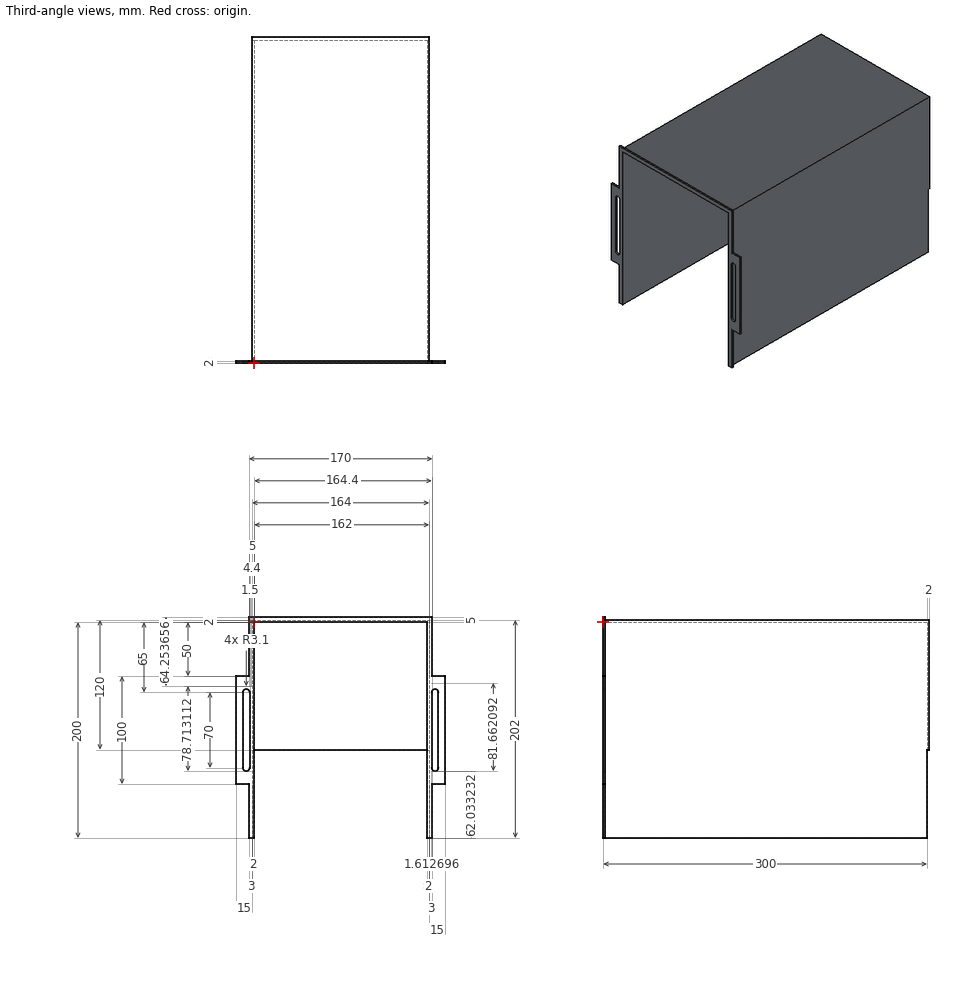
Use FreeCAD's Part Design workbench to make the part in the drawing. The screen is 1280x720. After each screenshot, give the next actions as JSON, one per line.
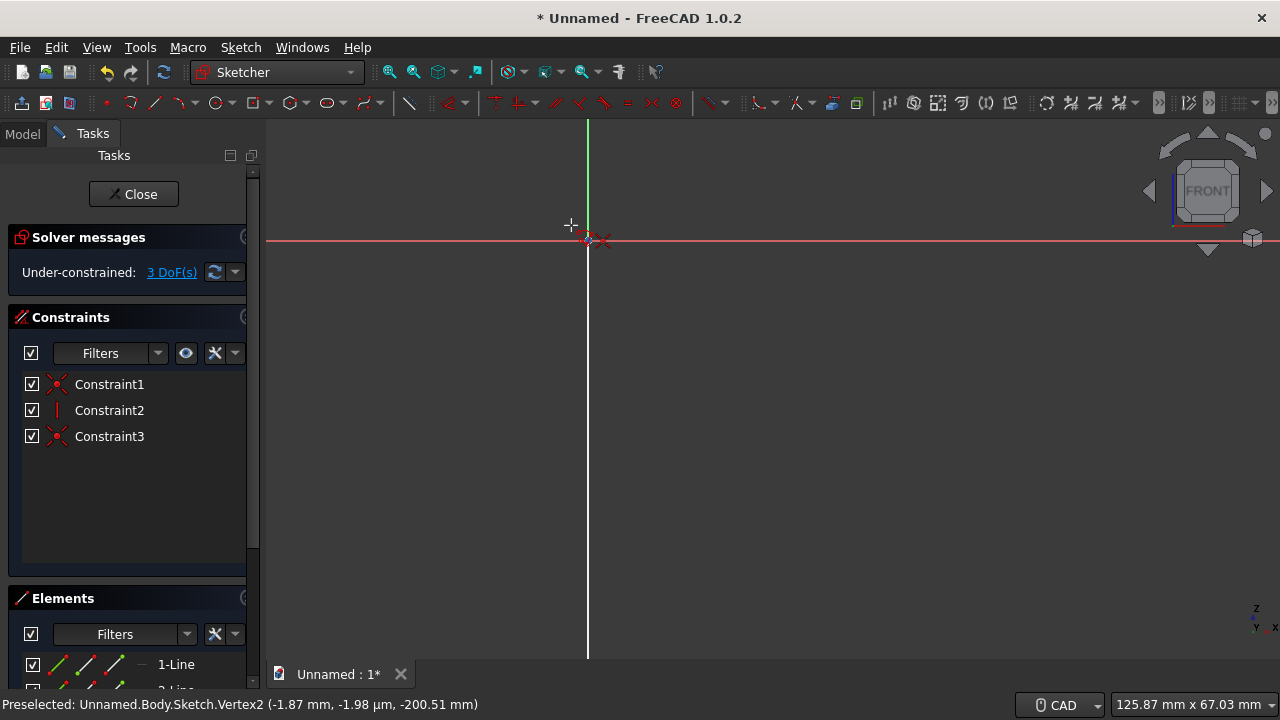
{"action": "left_click", "coordinate": [572, 225]}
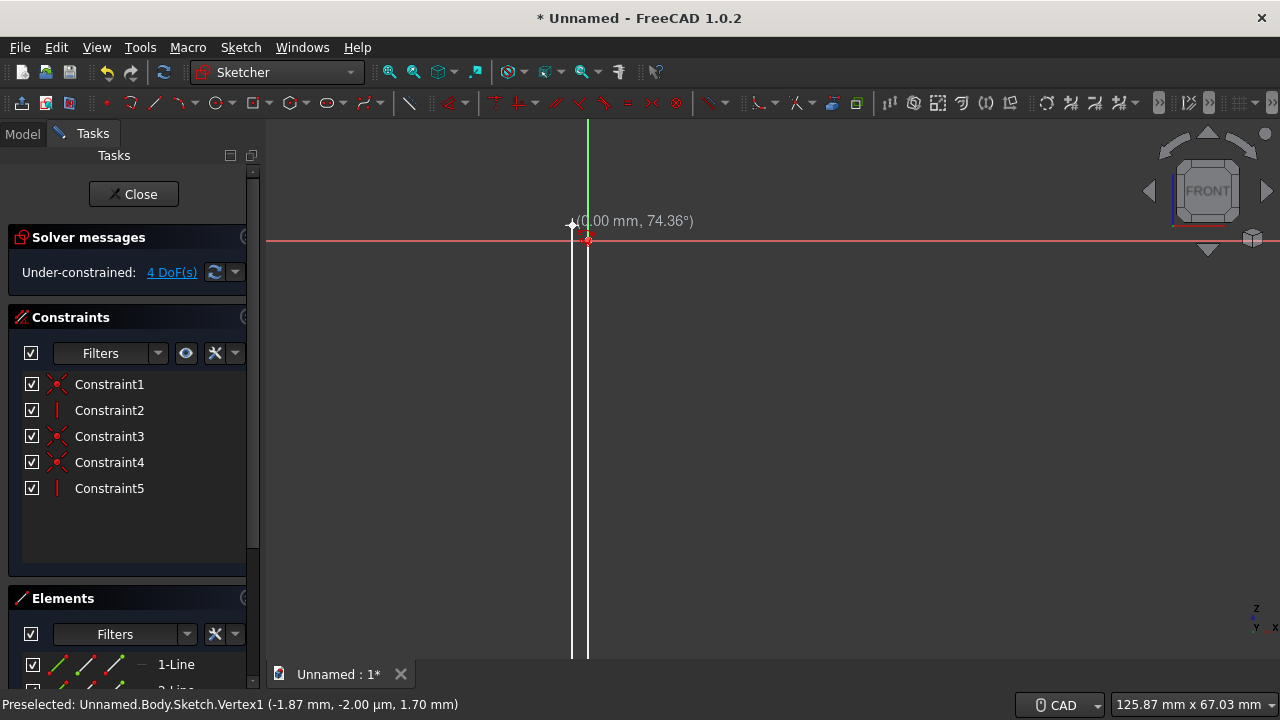
{"action": "scroll", "coordinate": [571, 225], "scroll_direction": "down", "scroll_amount": 8}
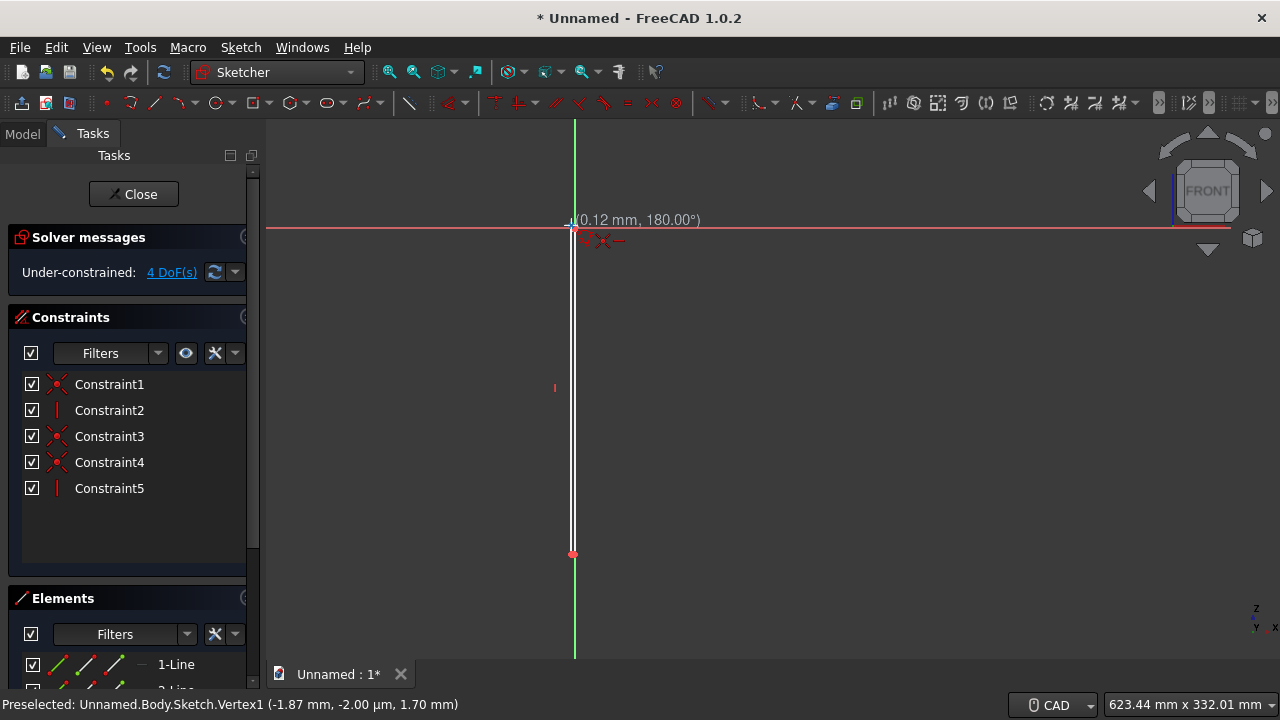
{"action": "scroll", "coordinate": [838, 225], "scroll_direction": "up", "scroll_amount": 8}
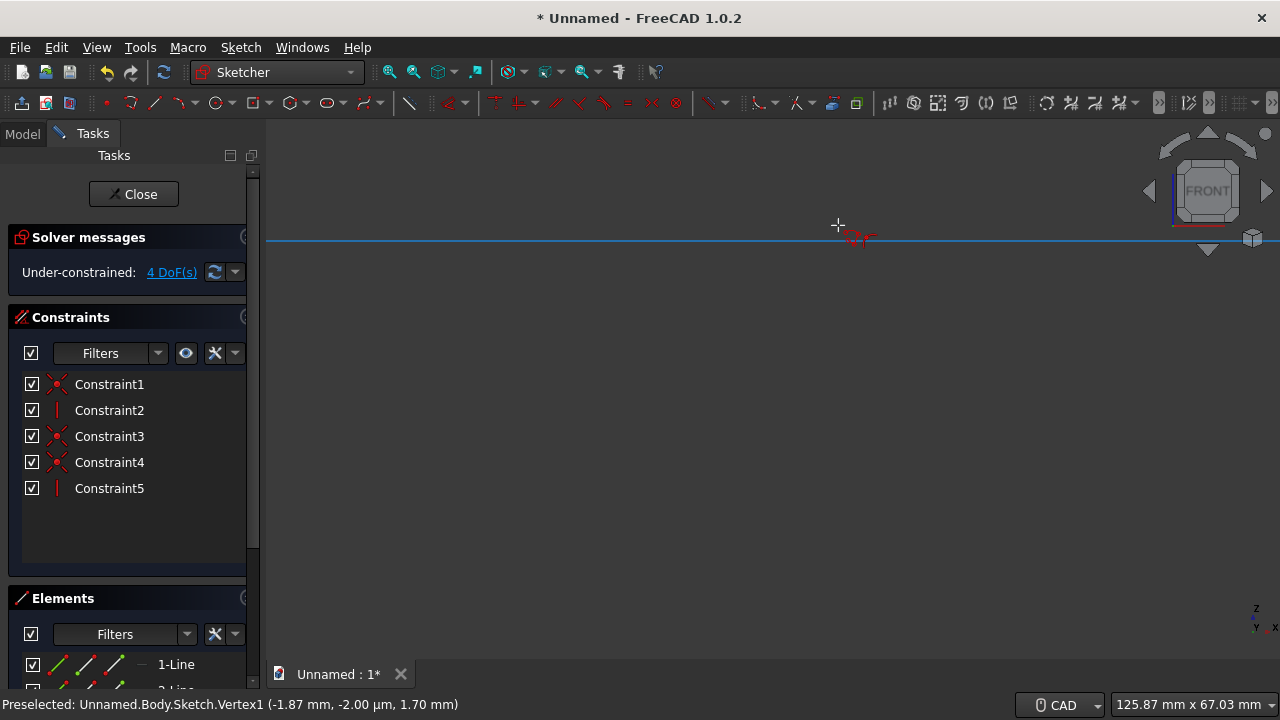
{"action": "left_click", "coordinate": [837, 225]}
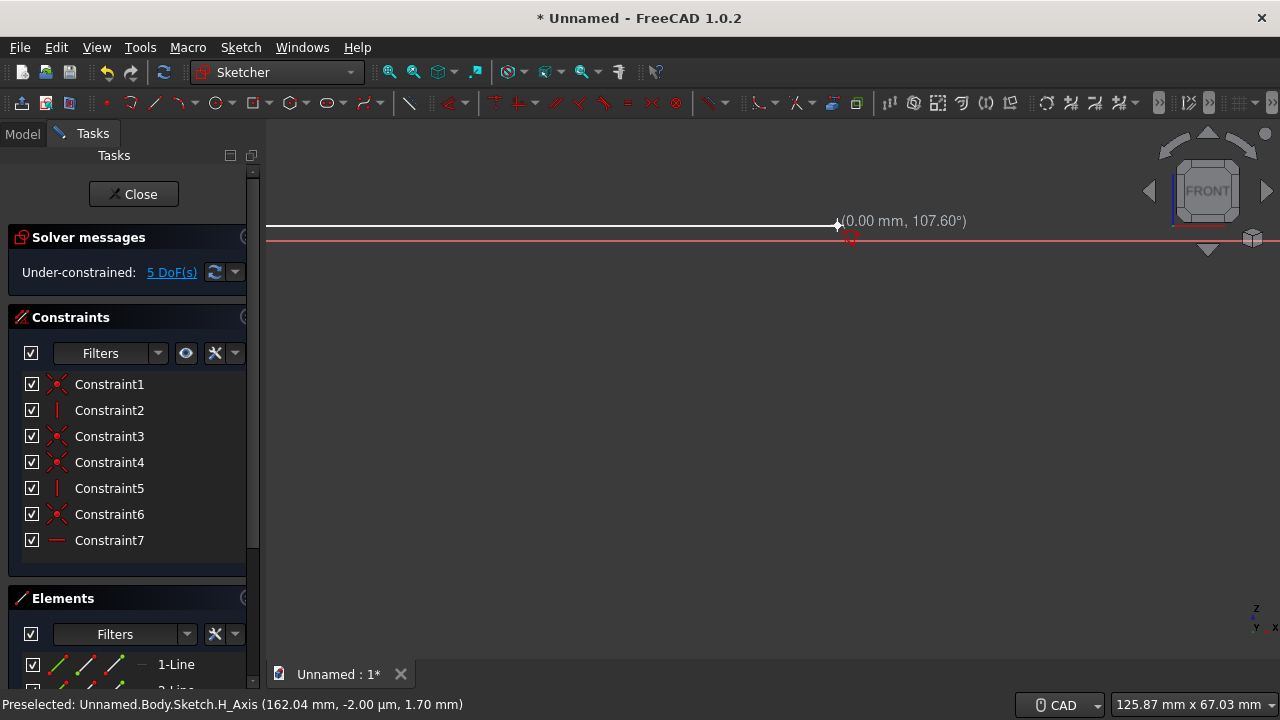
{"action": "scroll", "coordinate": [838, 225], "scroll_direction": "down", "scroll_amount": 8}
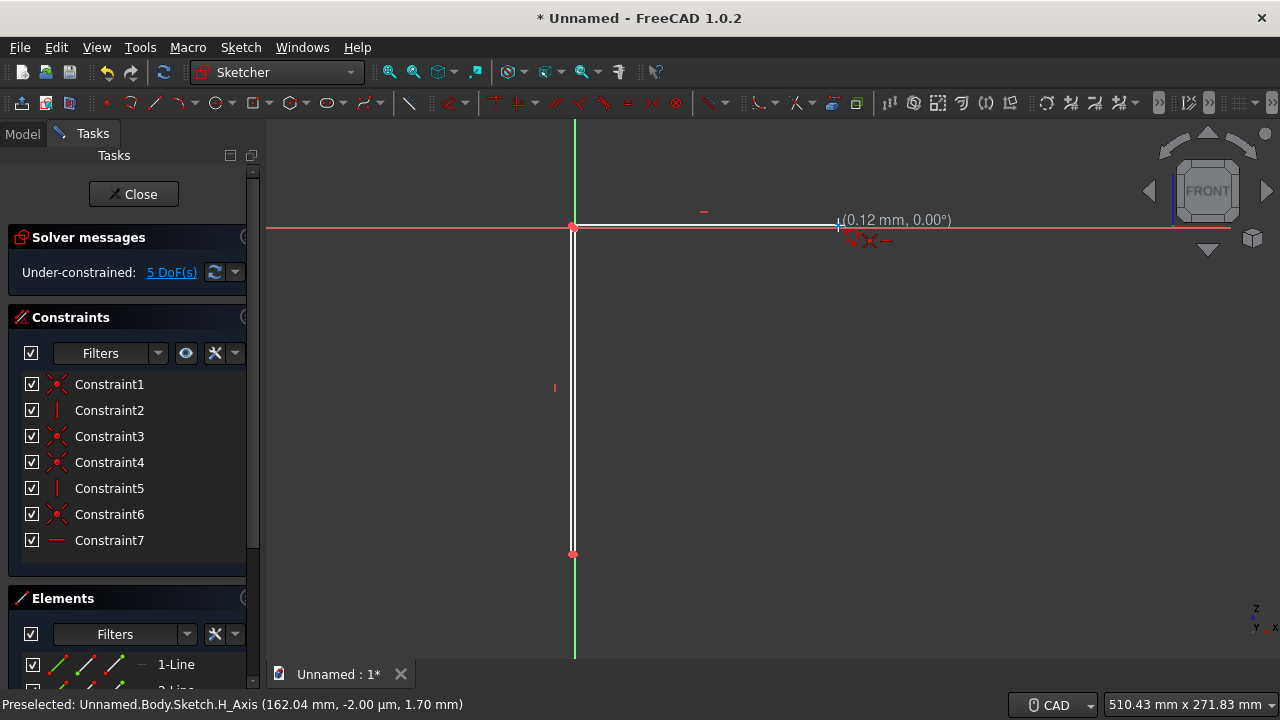
{"action": "left_click", "coordinate": [838, 554]}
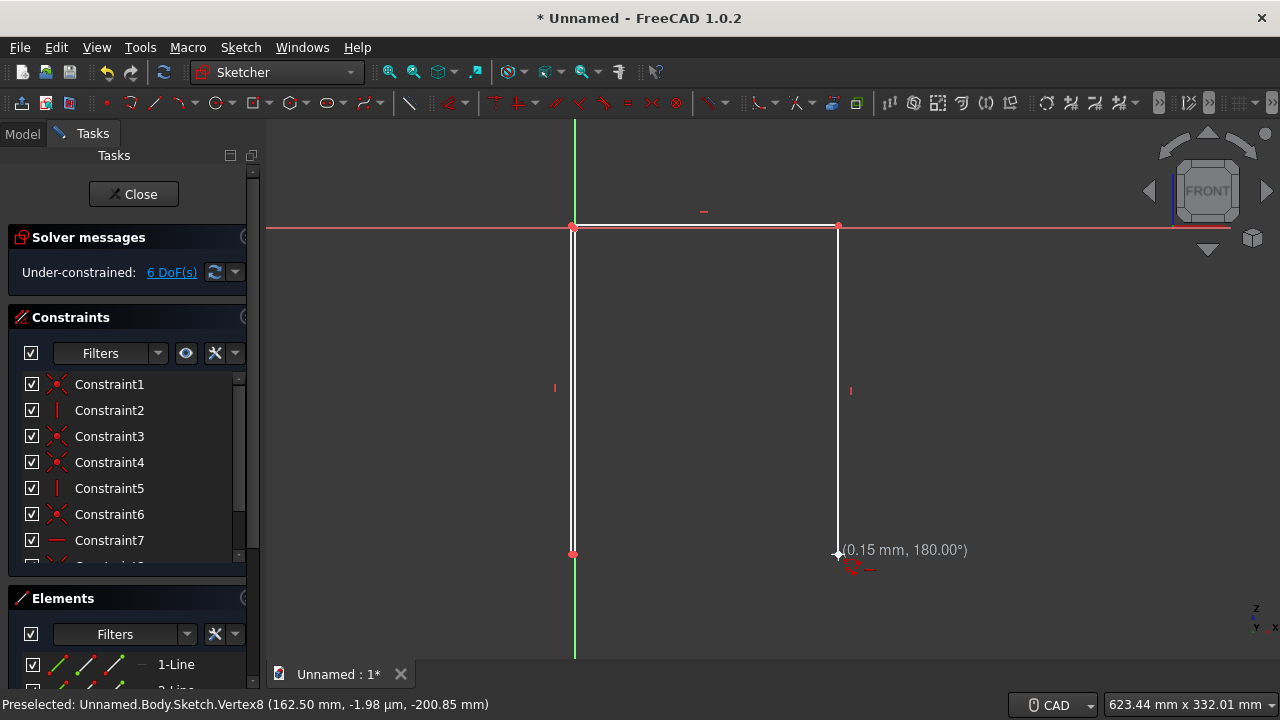
{"action": "scroll", "coordinate": [835, 554], "scroll_direction": "up", "scroll_amount": 8}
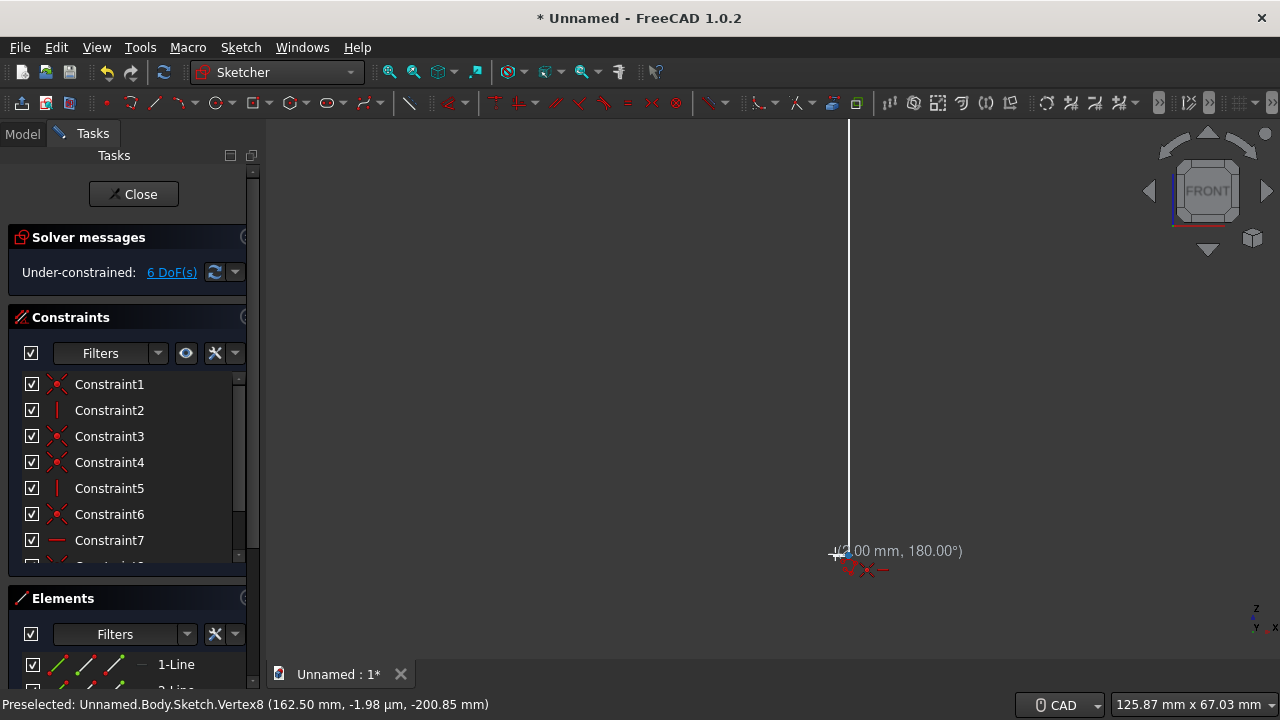
{"action": "left_click", "coordinate": [832, 551]}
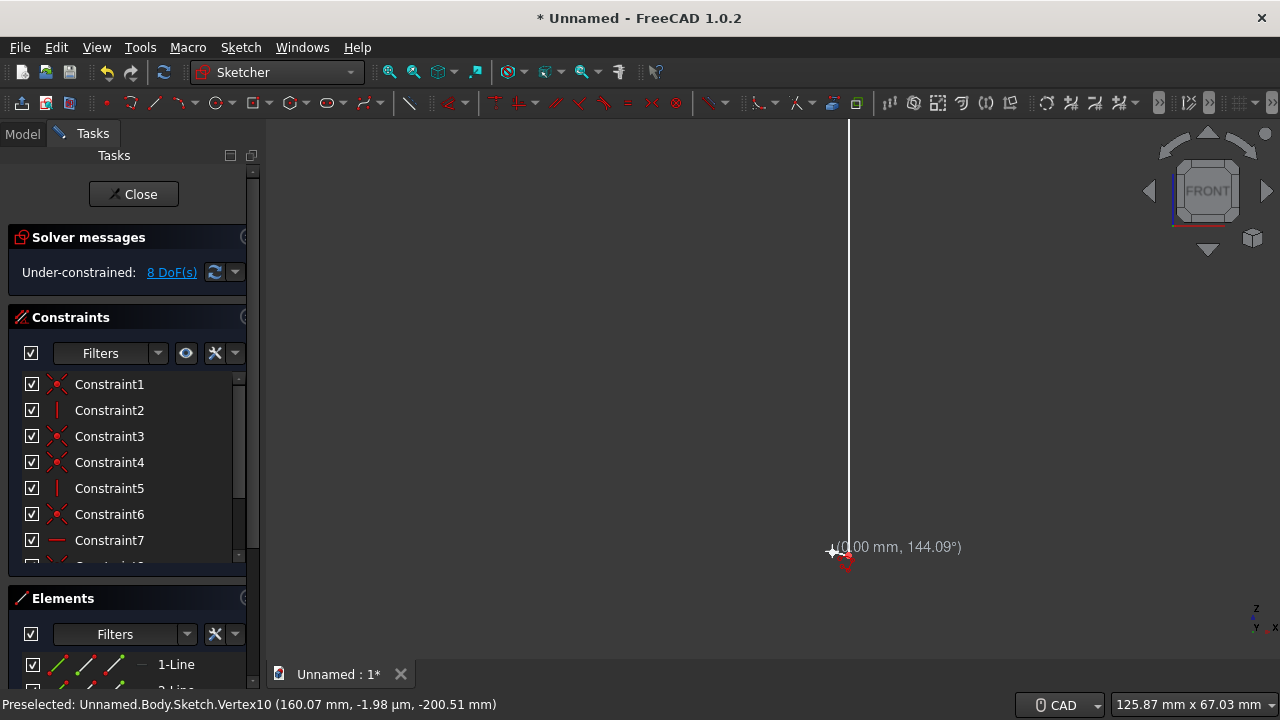
{"action": "scroll", "coordinate": [835, 554], "scroll_direction": "down", "scroll_amount": 8}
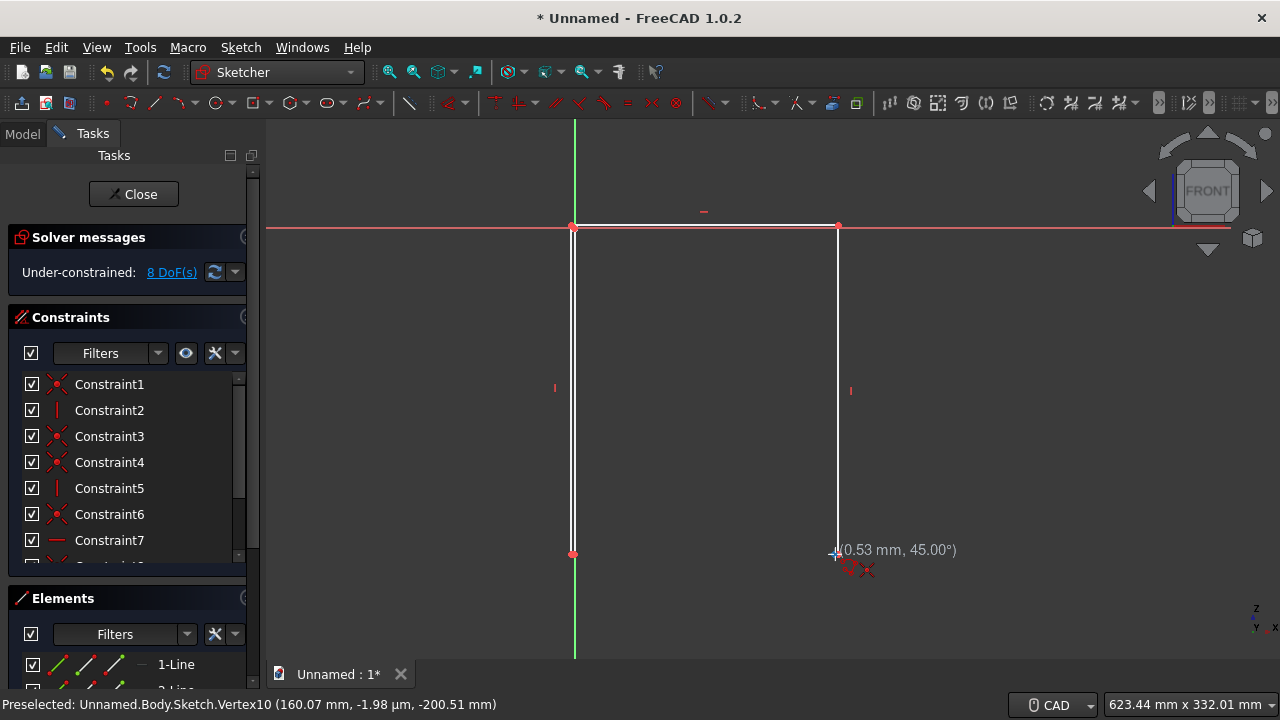
{"action": "scroll", "coordinate": [835, 228], "scroll_direction": "up", "scroll_amount": 8}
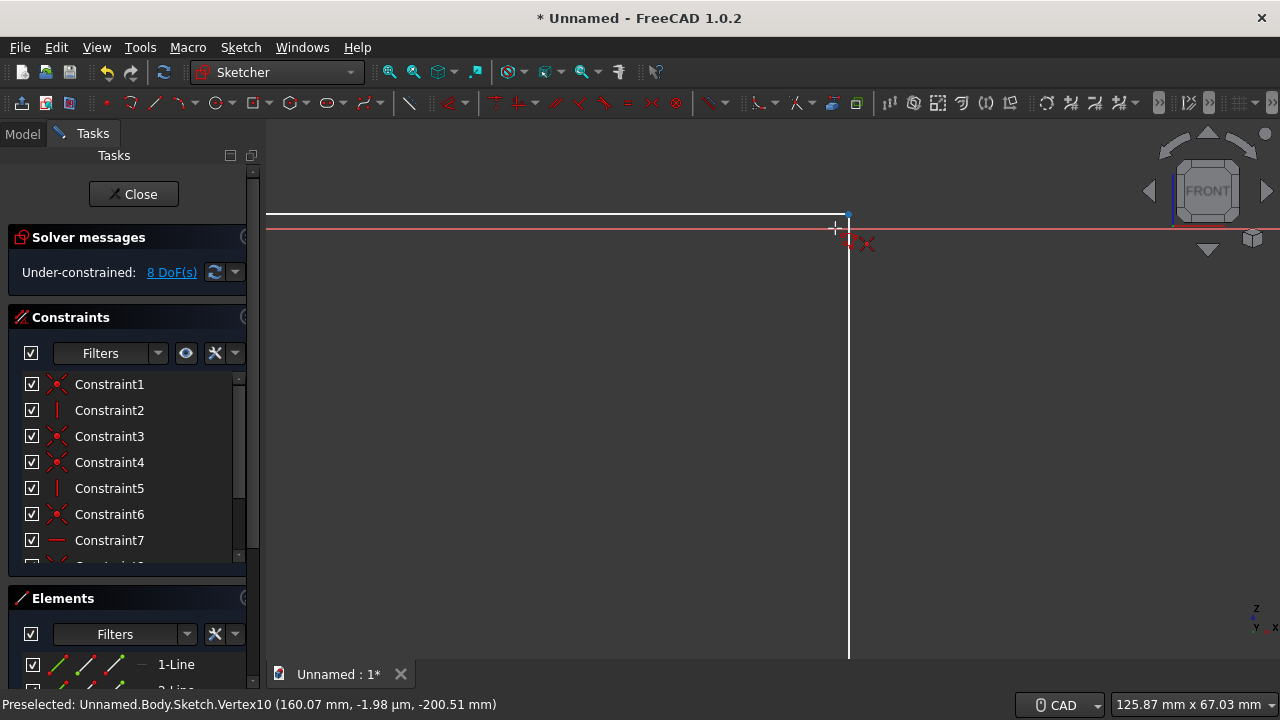
{"action": "left_click", "coordinate": [832, 238]}